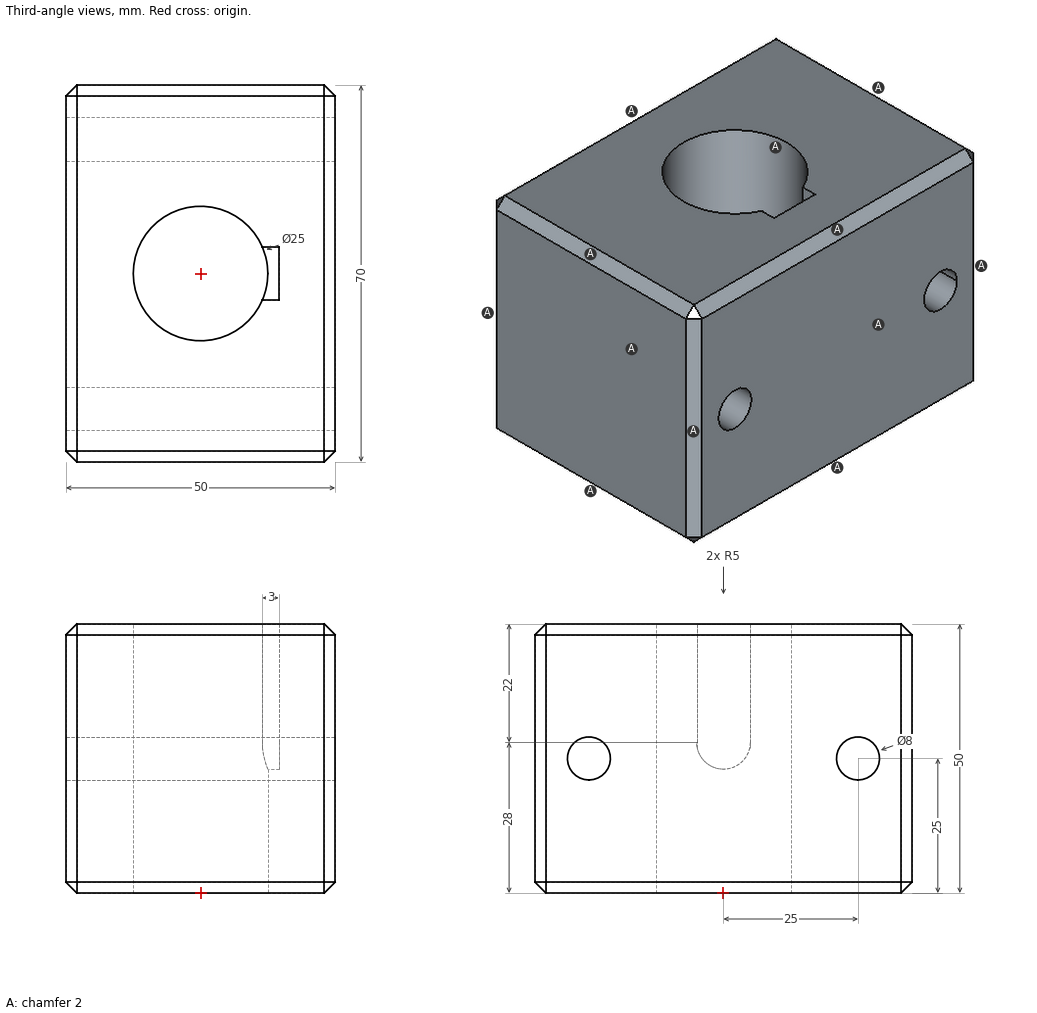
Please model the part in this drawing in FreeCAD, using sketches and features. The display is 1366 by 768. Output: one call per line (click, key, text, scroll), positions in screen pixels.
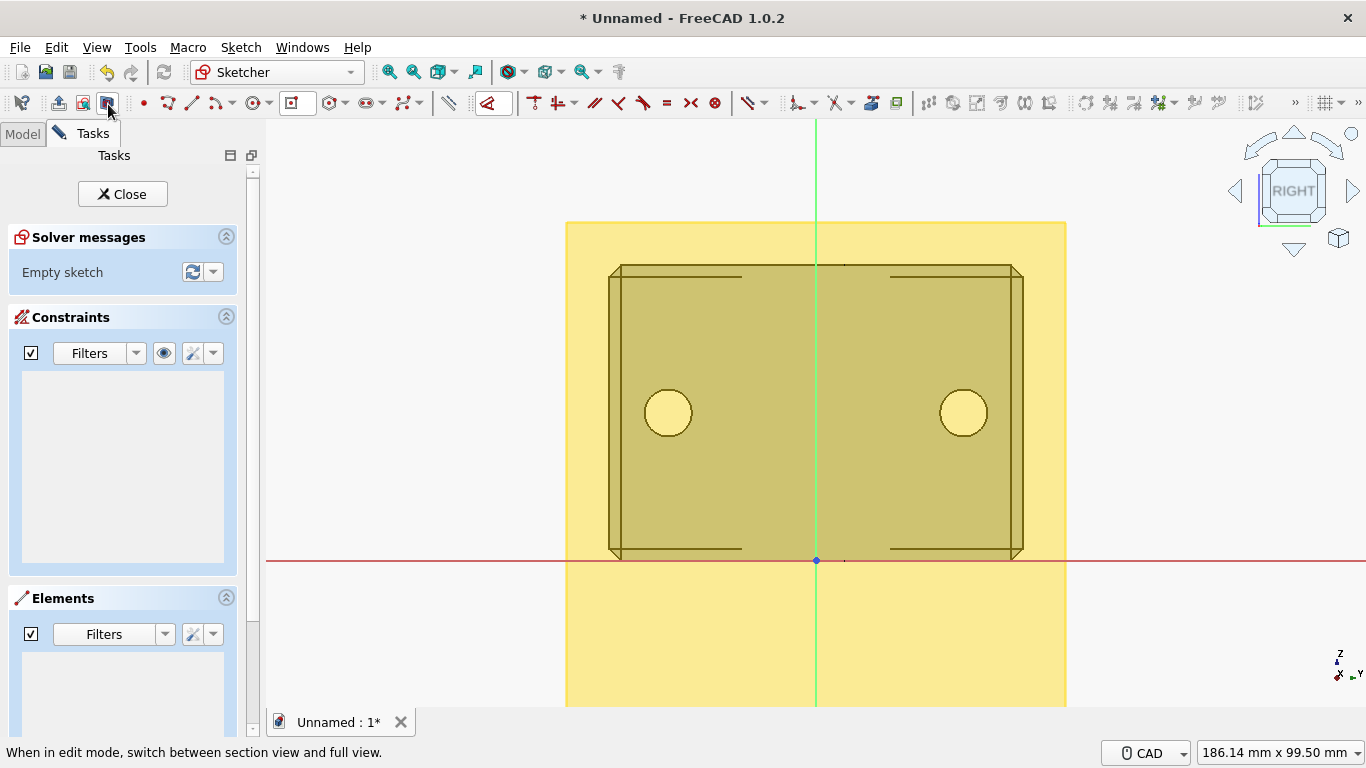
click(366, 104)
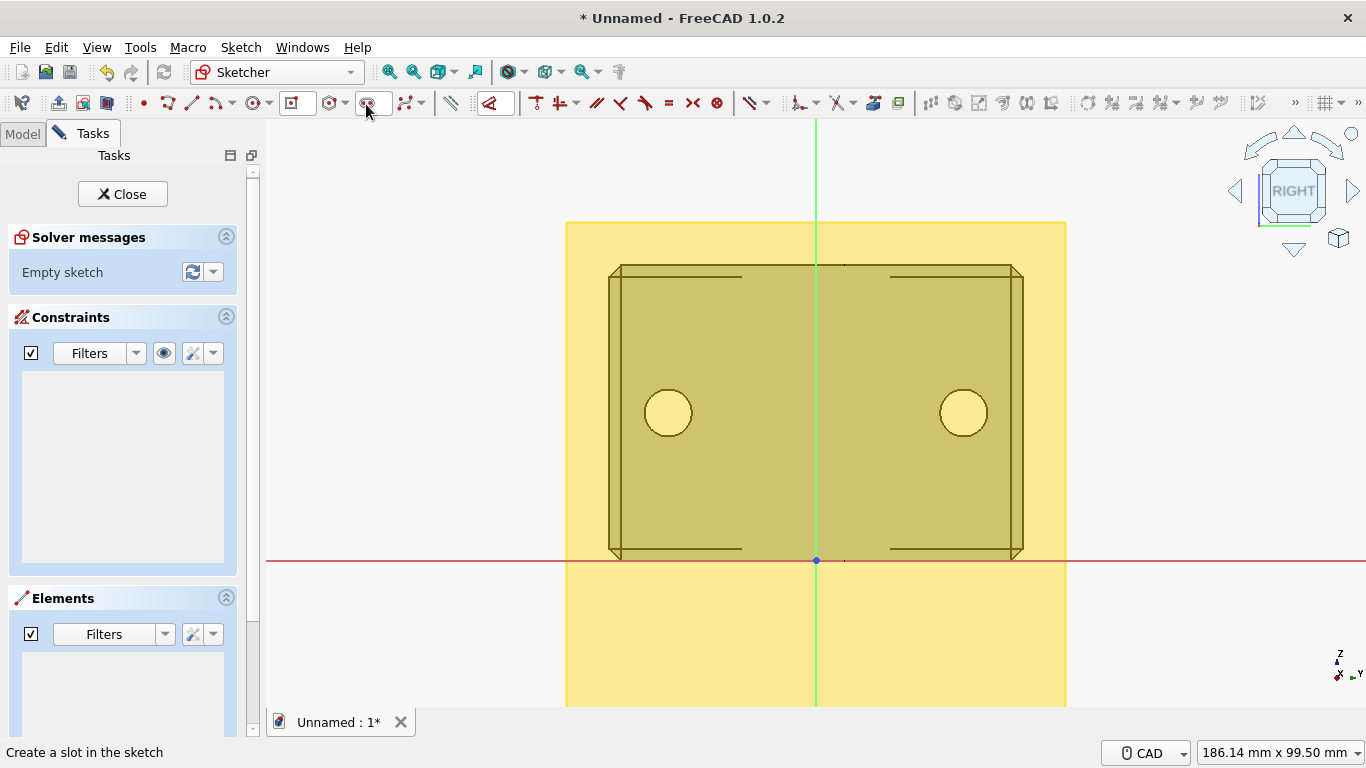
click(816, 395)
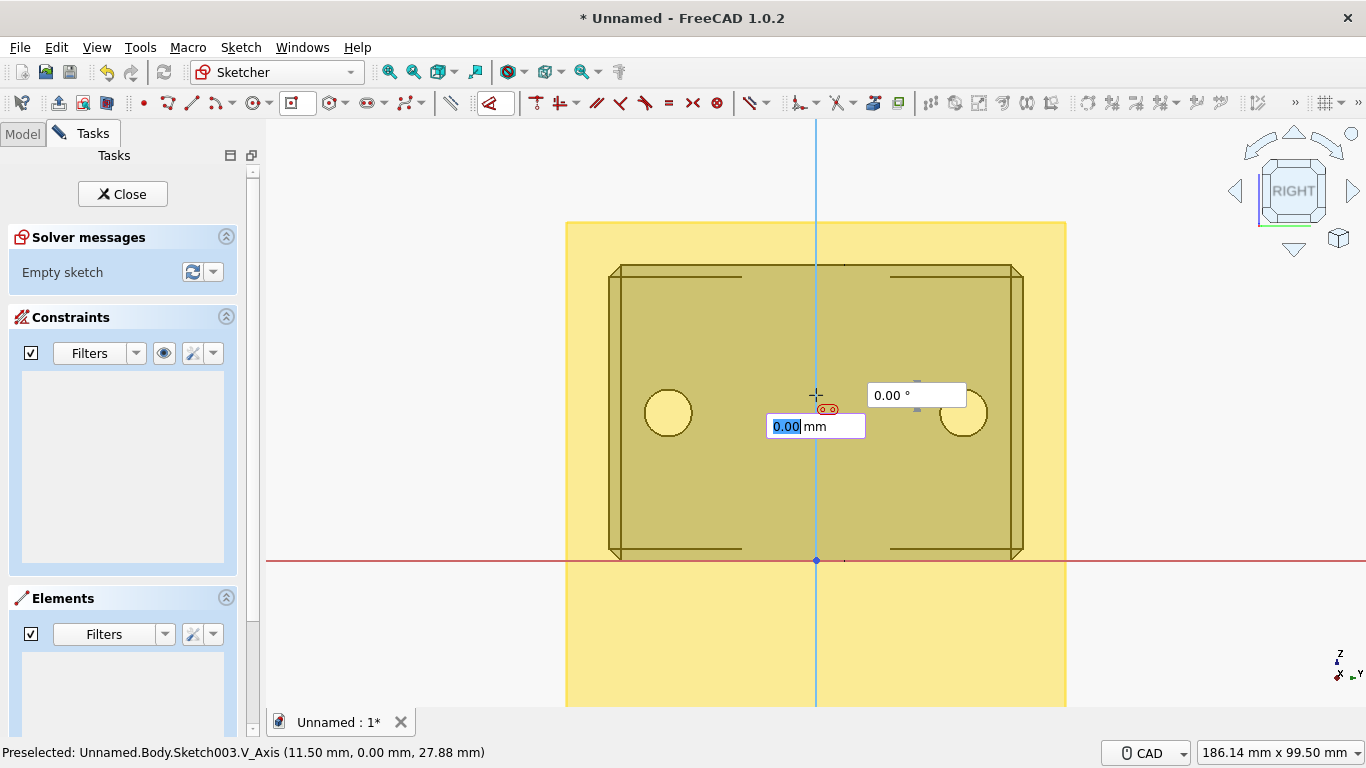
click(825, 265)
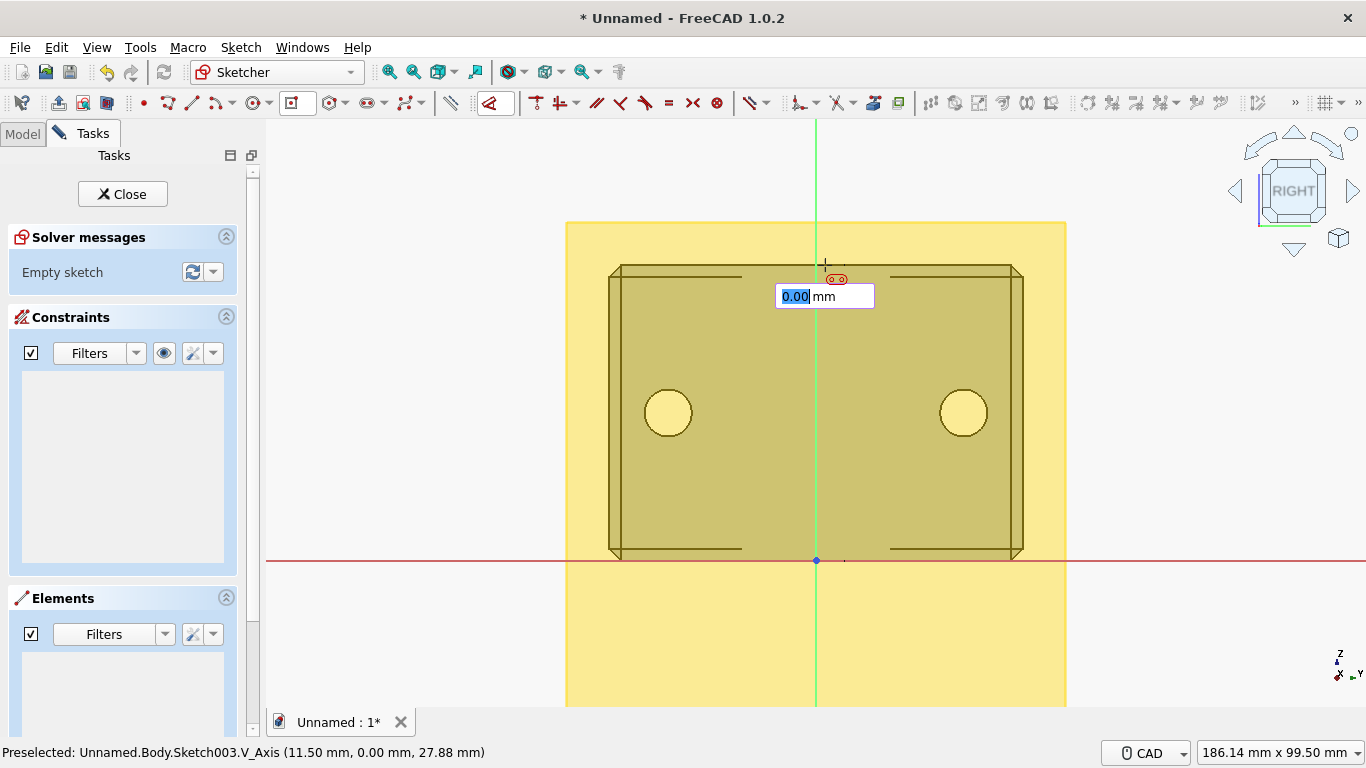
click(846, 330)
key(Escape)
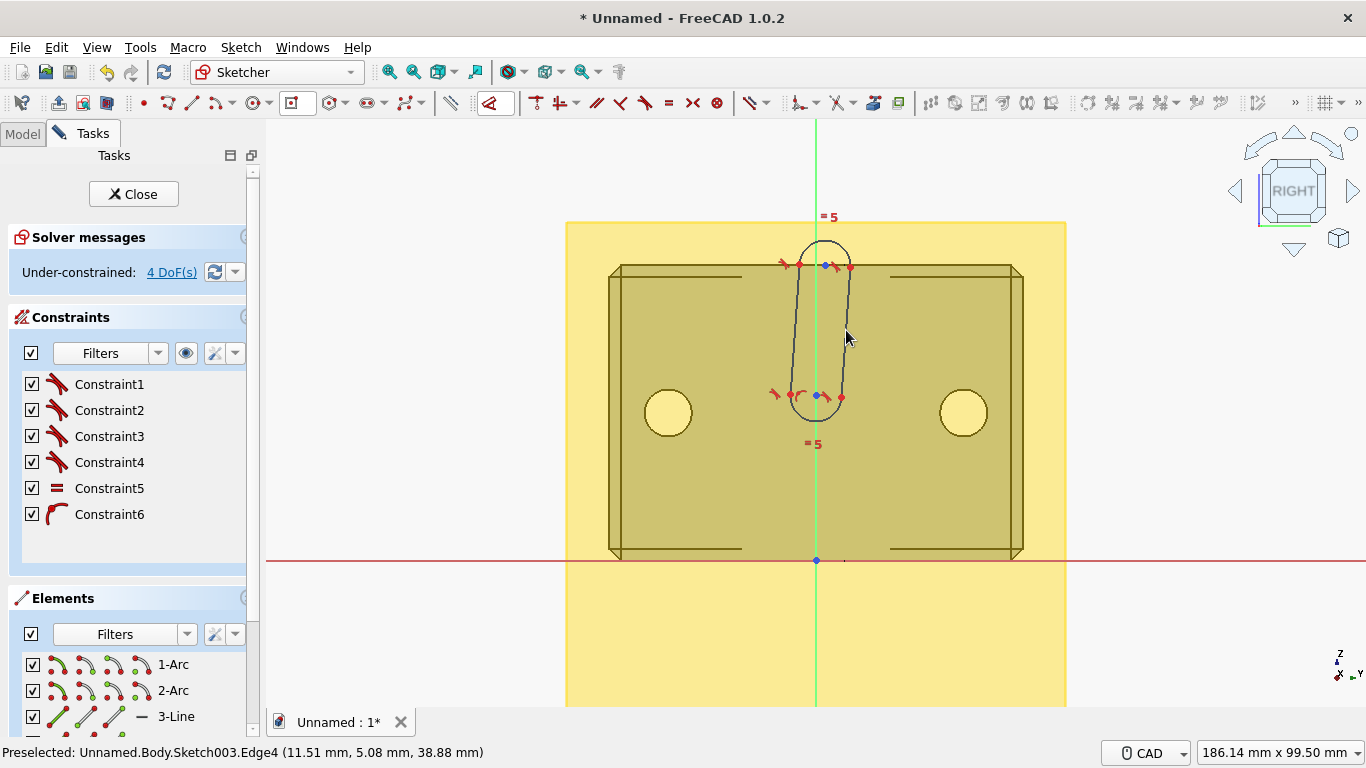
click(793, 355)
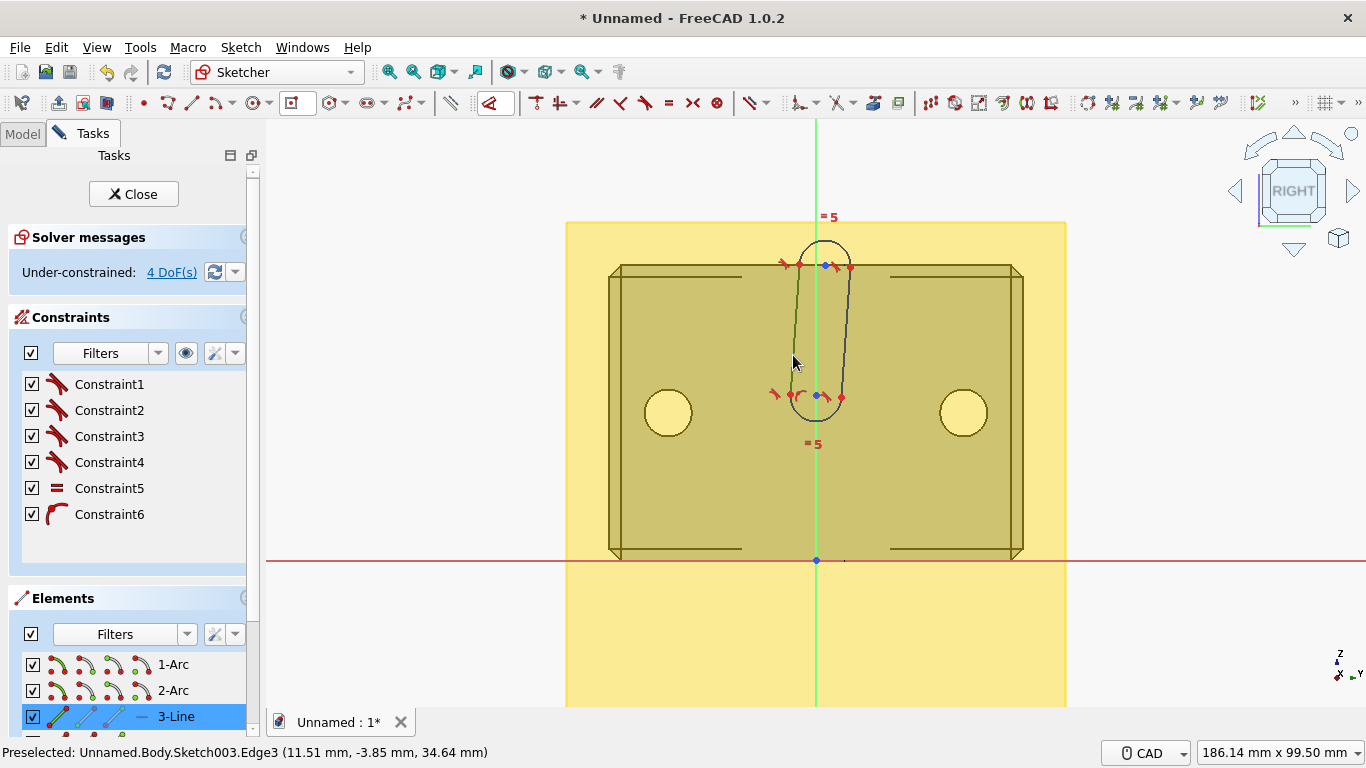
key(v)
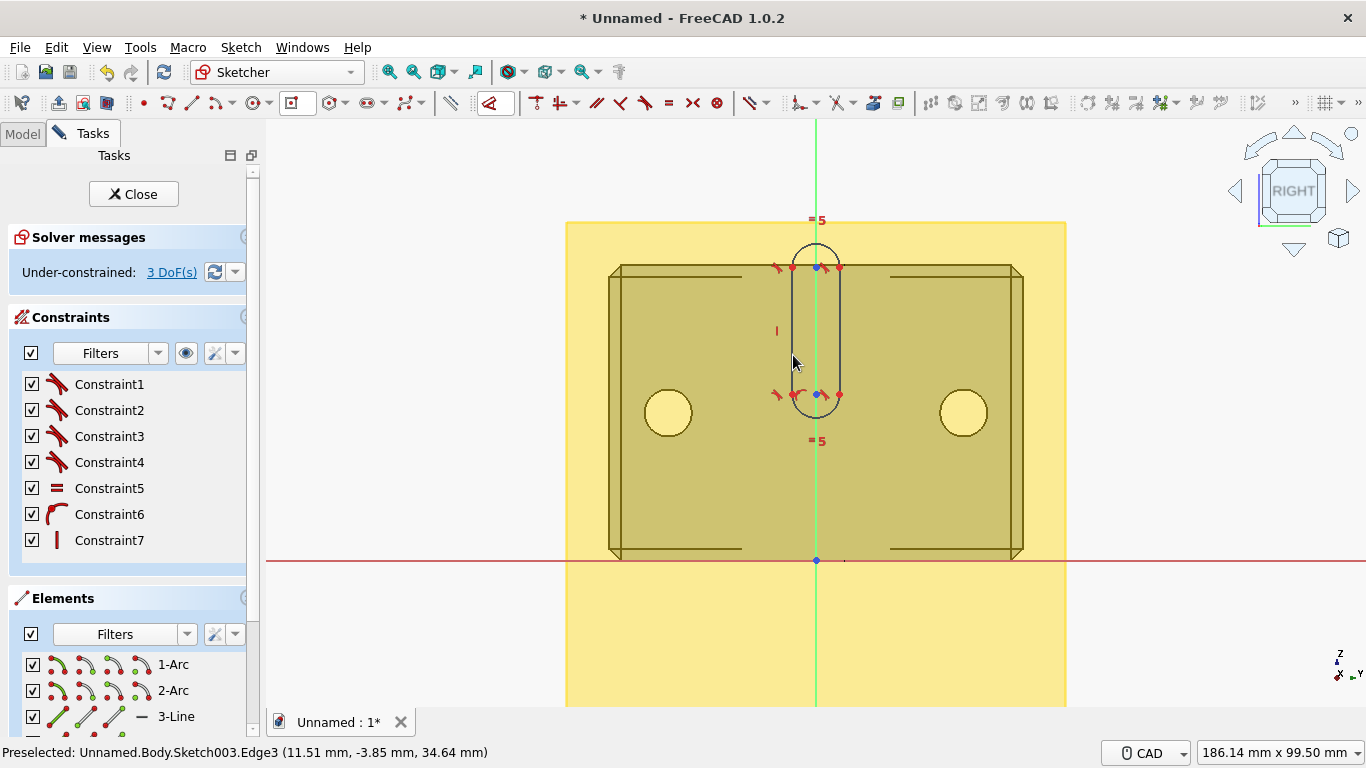
scroll(802, 413, up, 2)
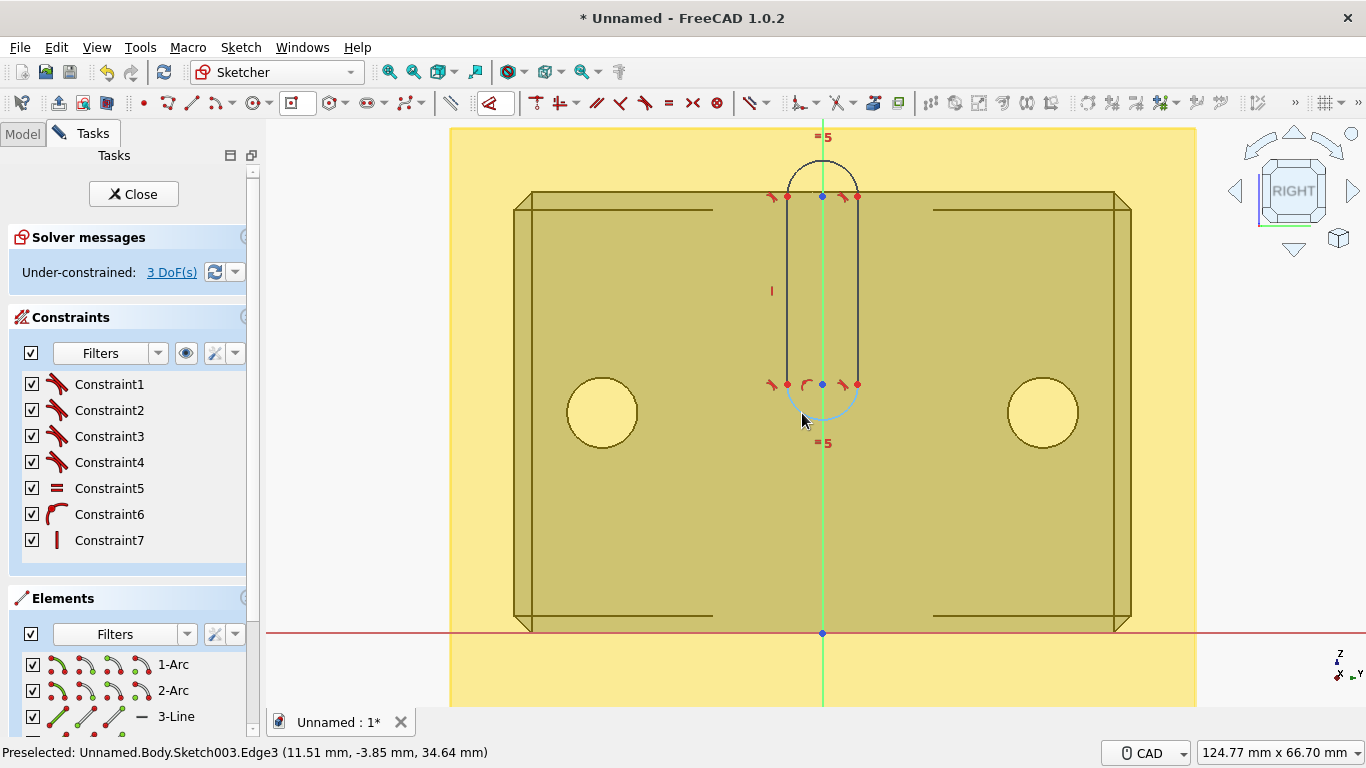
click(802, 413)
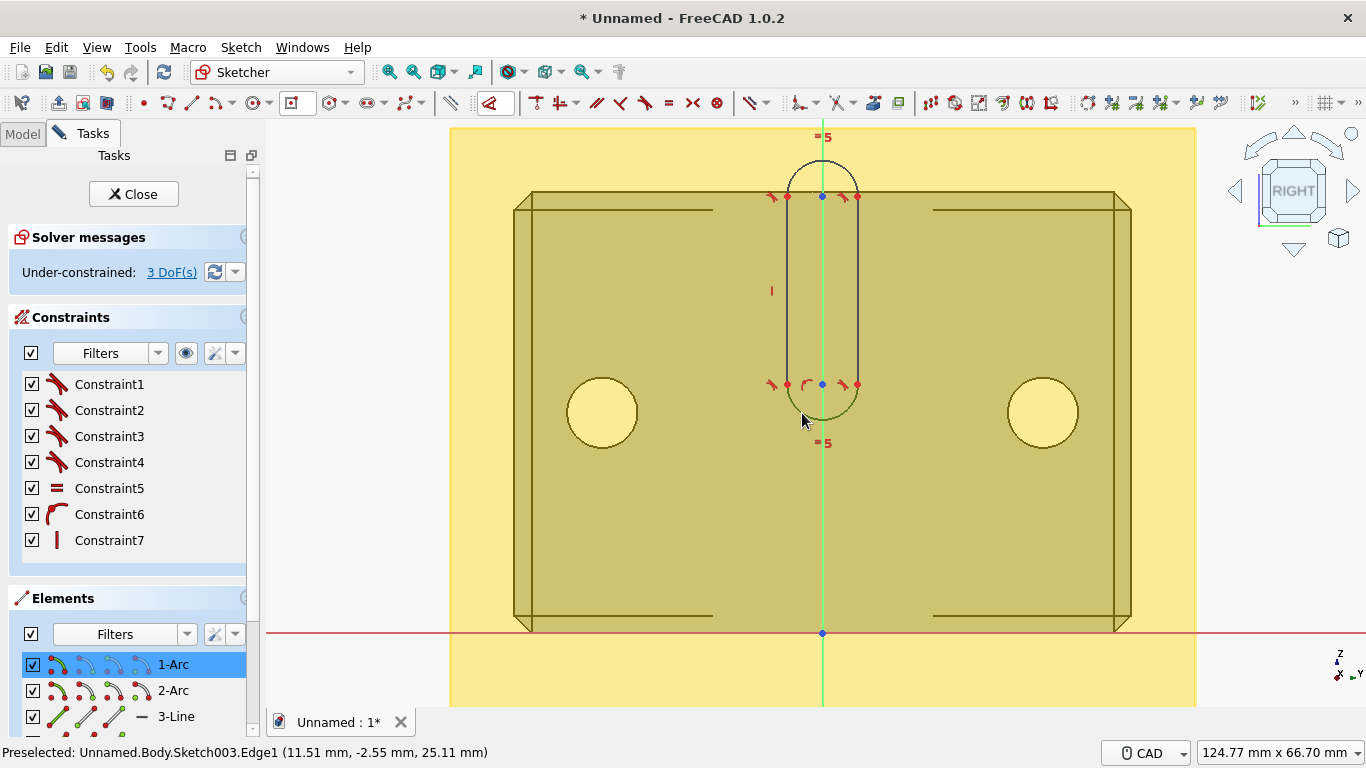
key(k)
key(r)